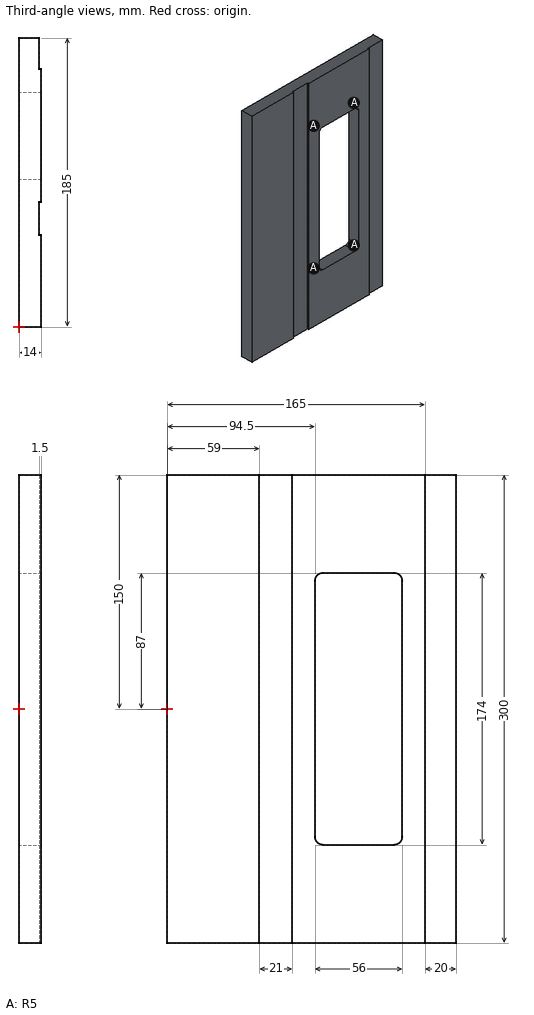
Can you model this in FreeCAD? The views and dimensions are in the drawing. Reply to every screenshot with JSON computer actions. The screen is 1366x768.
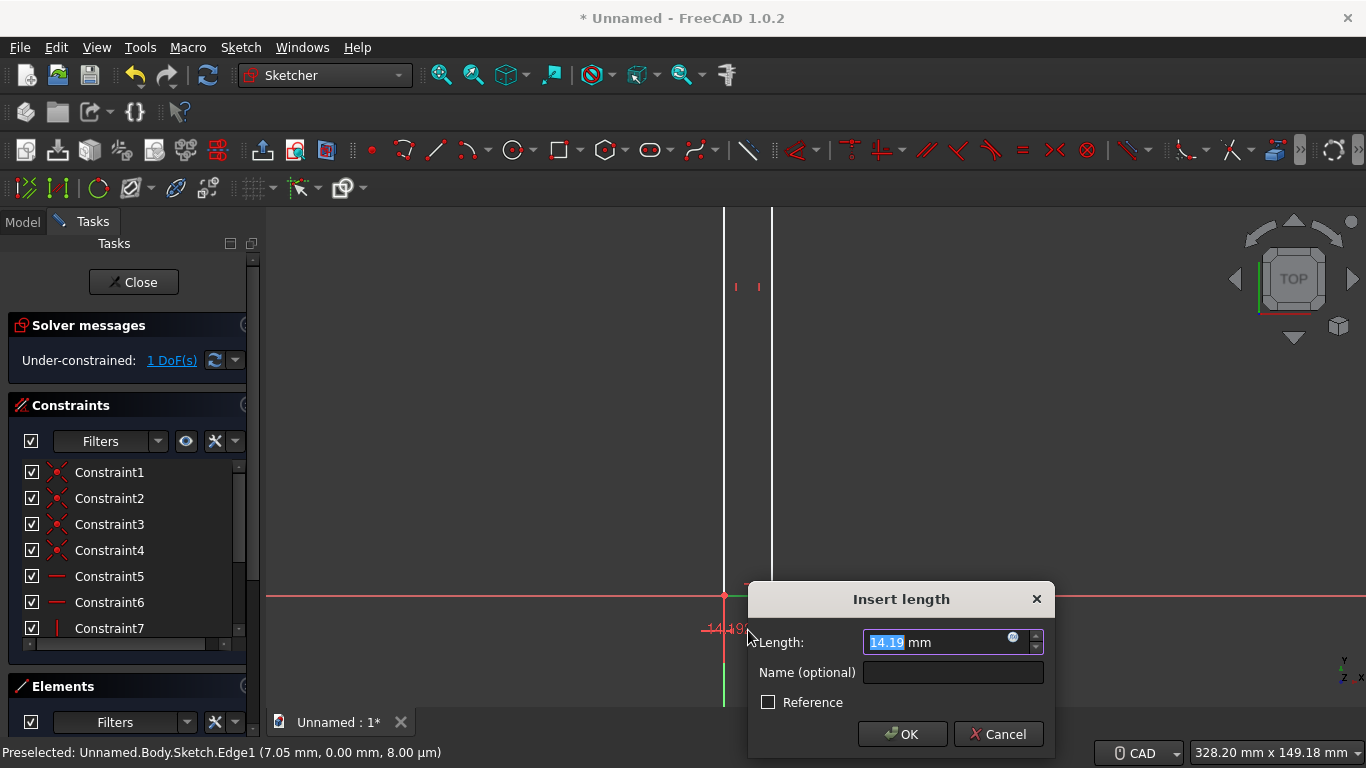
{"action": "type", "text": "14"}
{"action": "key", "text": "Return"}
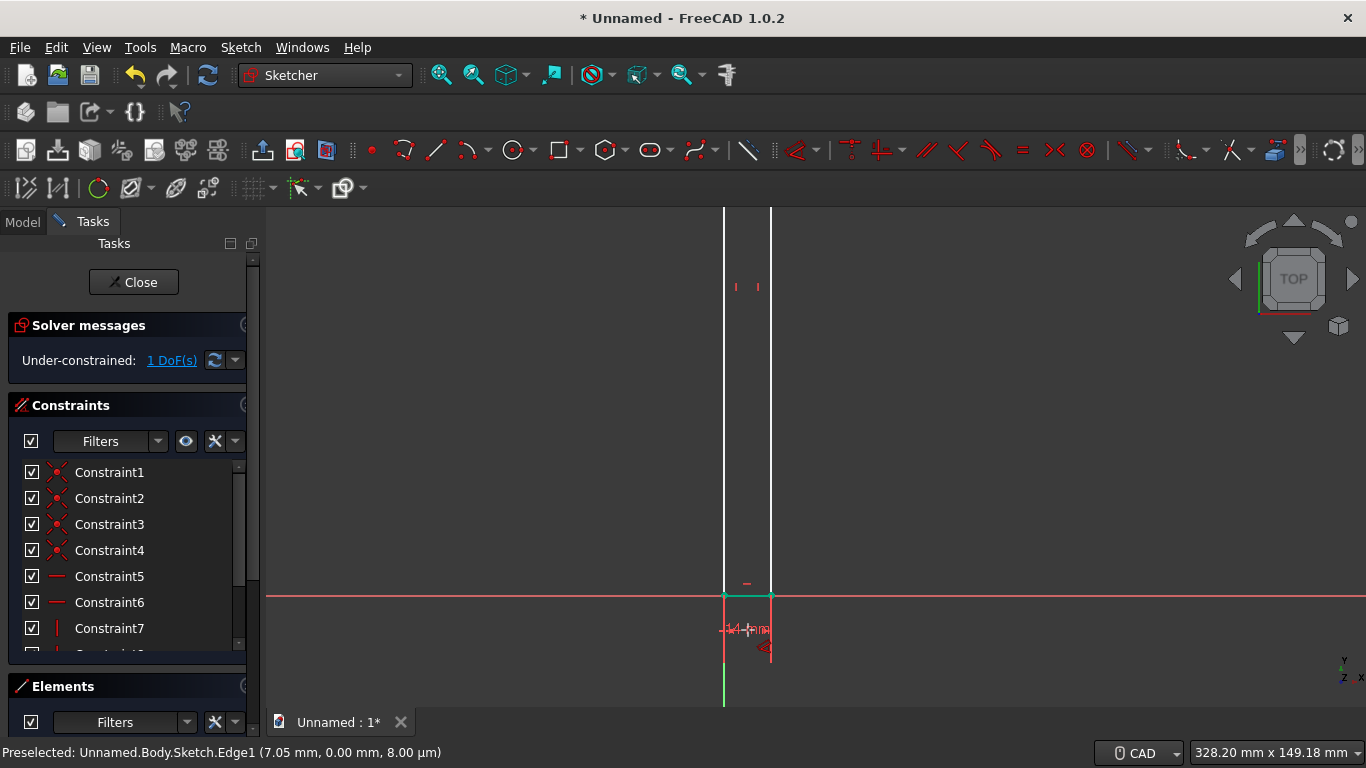
{"action": "left_click", "coordinate": [771, 410]}
{"action": "left_click", "coordinate": [805, 415]}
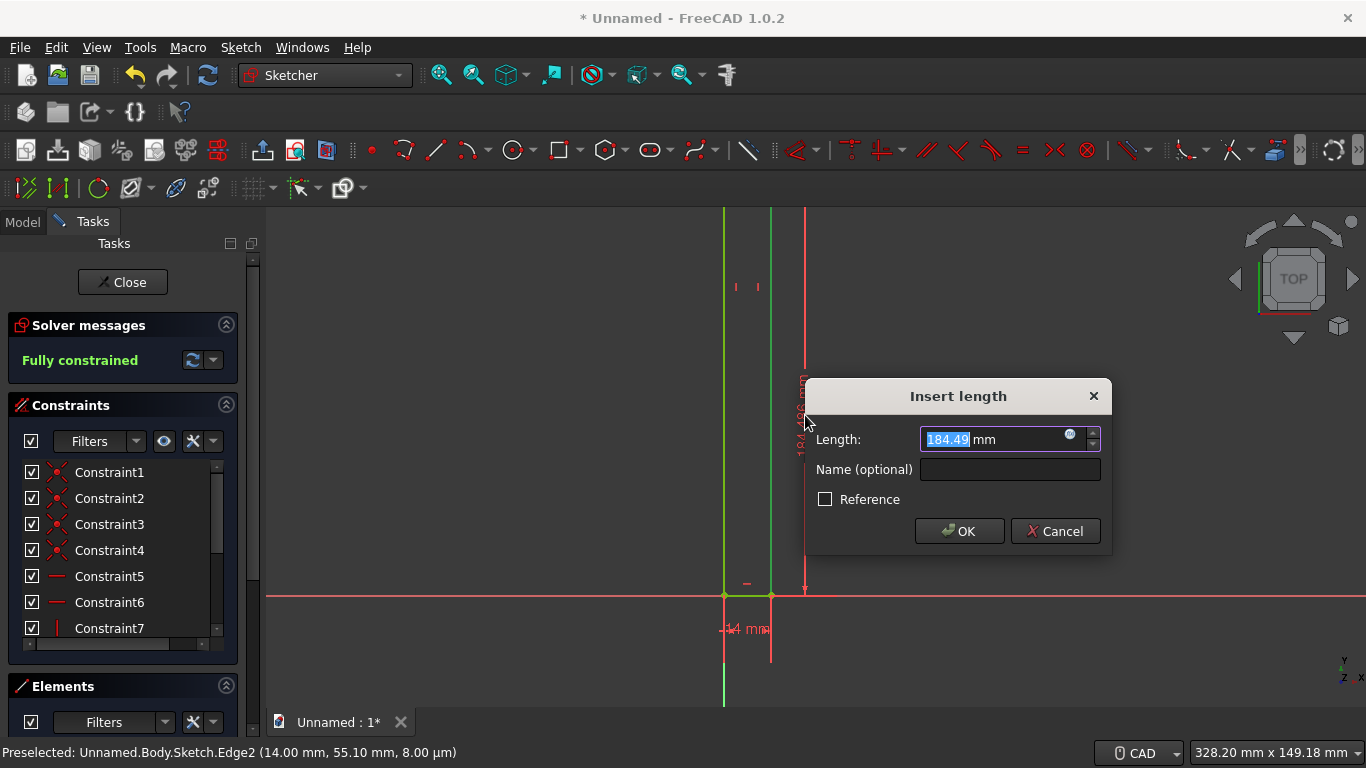
{"action": "type", "text": "185"}
{"action": "key", "text": "Return"}
{"action": "key", "text": "Escape"}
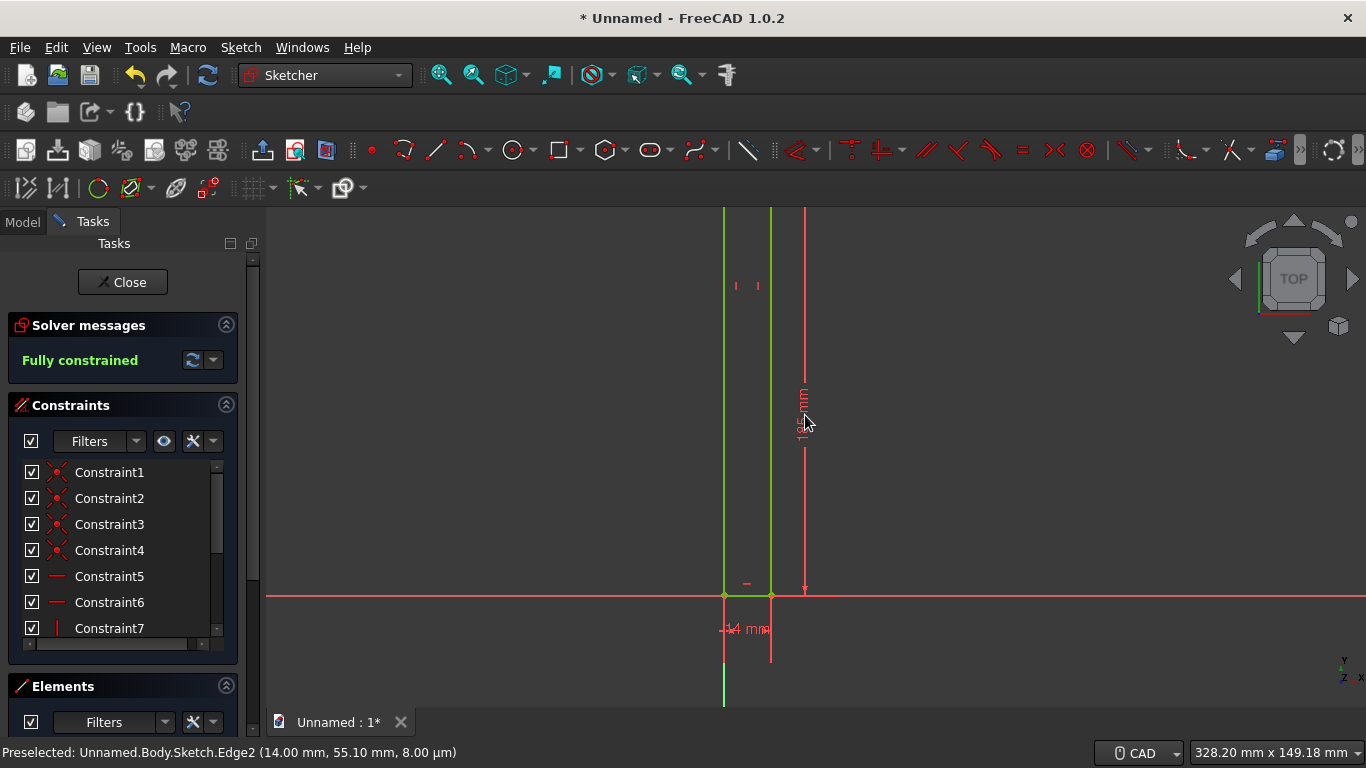
{"action": "left_click", "coordinate": [123, 282]}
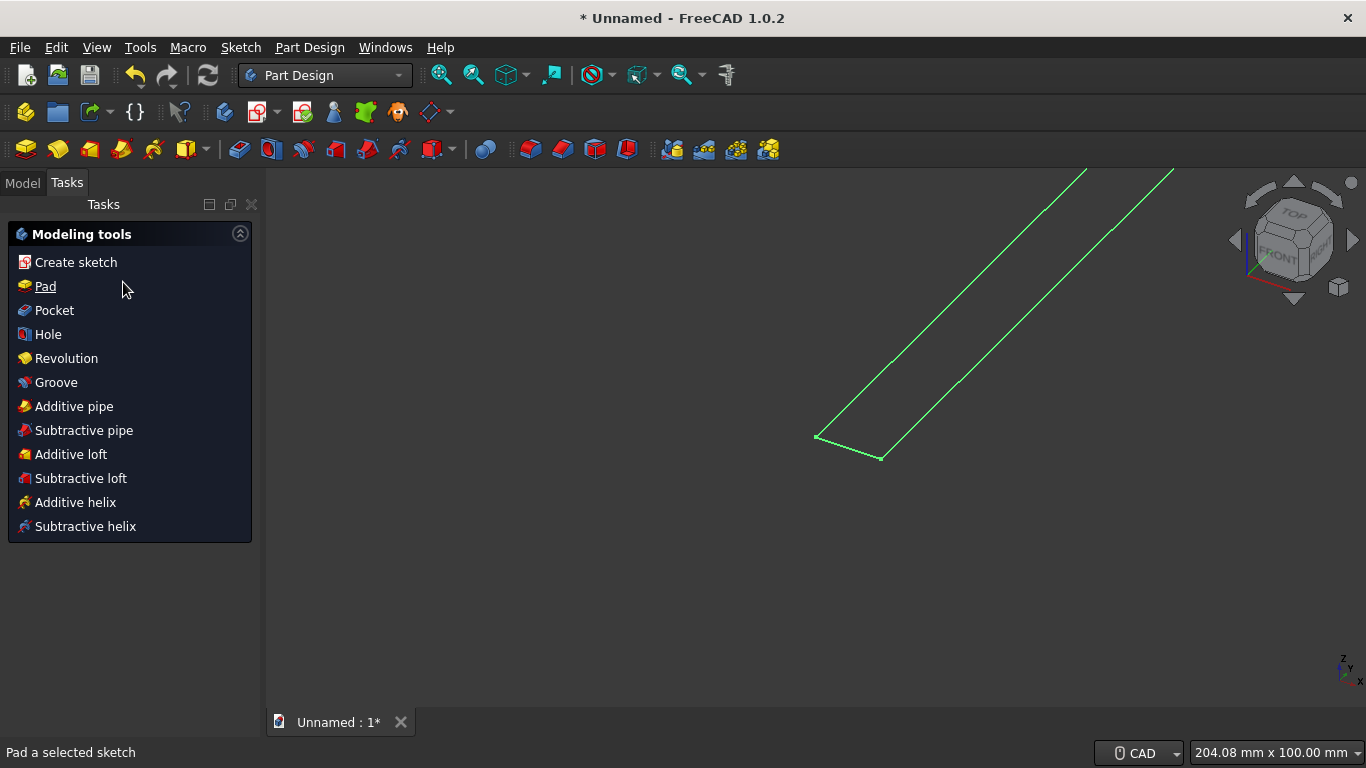
{"action": "left_click", "coordinate": [26, 150]}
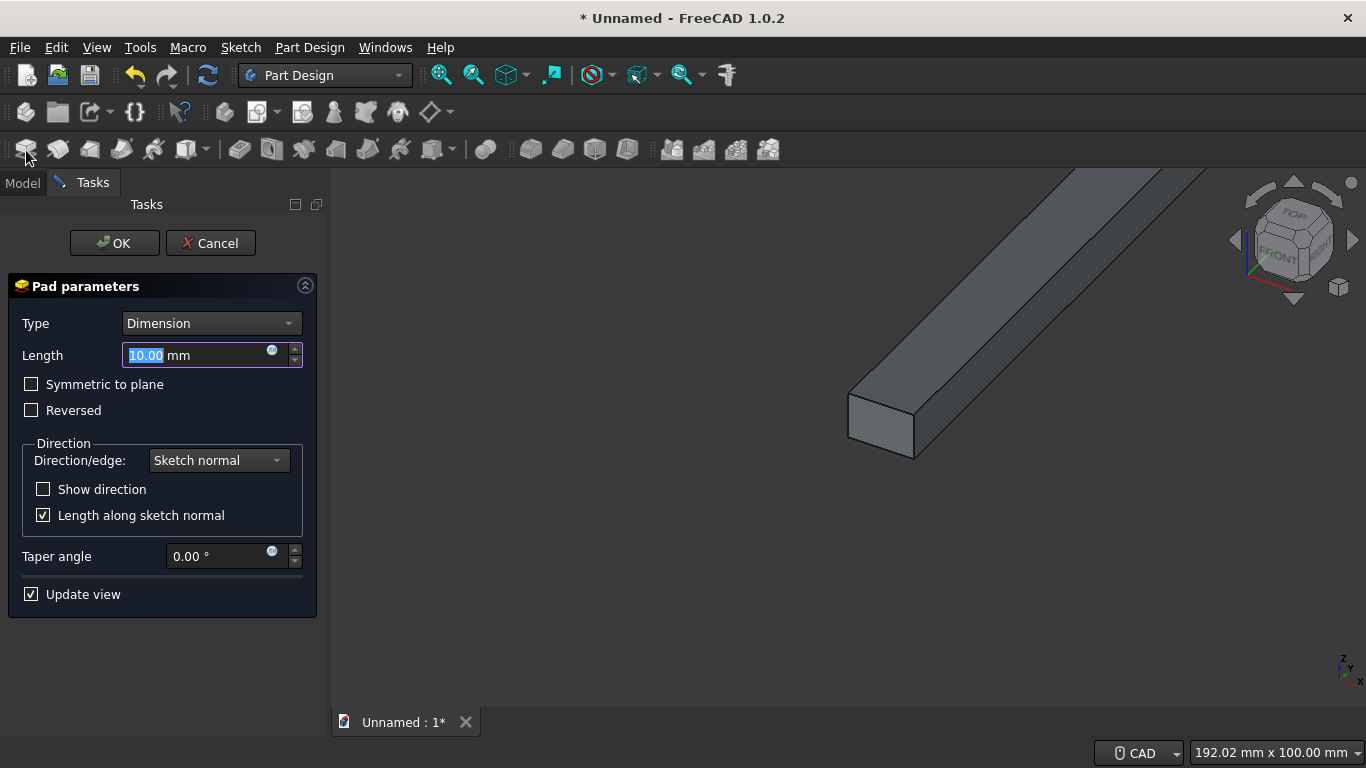
{"action": "type", "text": "300"}
{"action": "key", "text": "Tab"}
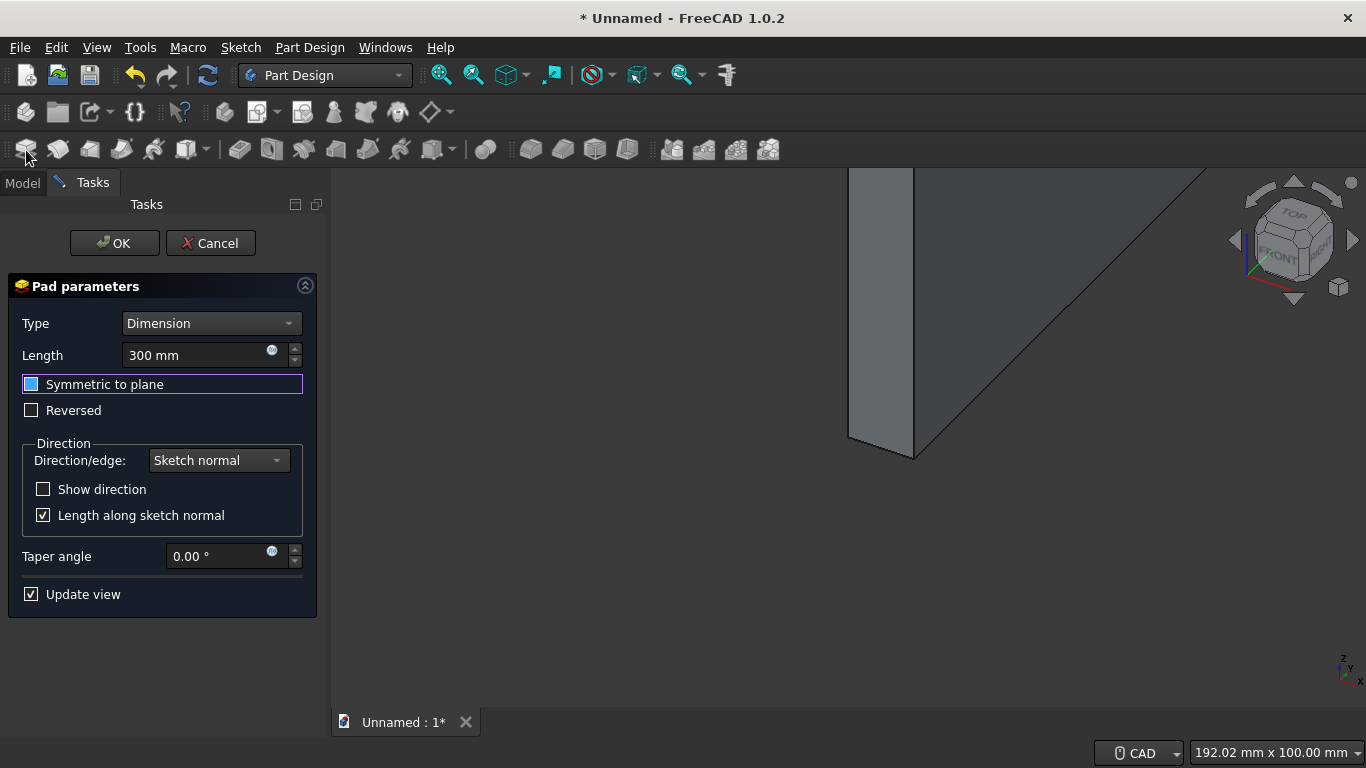
{"action": "left_click", "coordinate": [30, 384]}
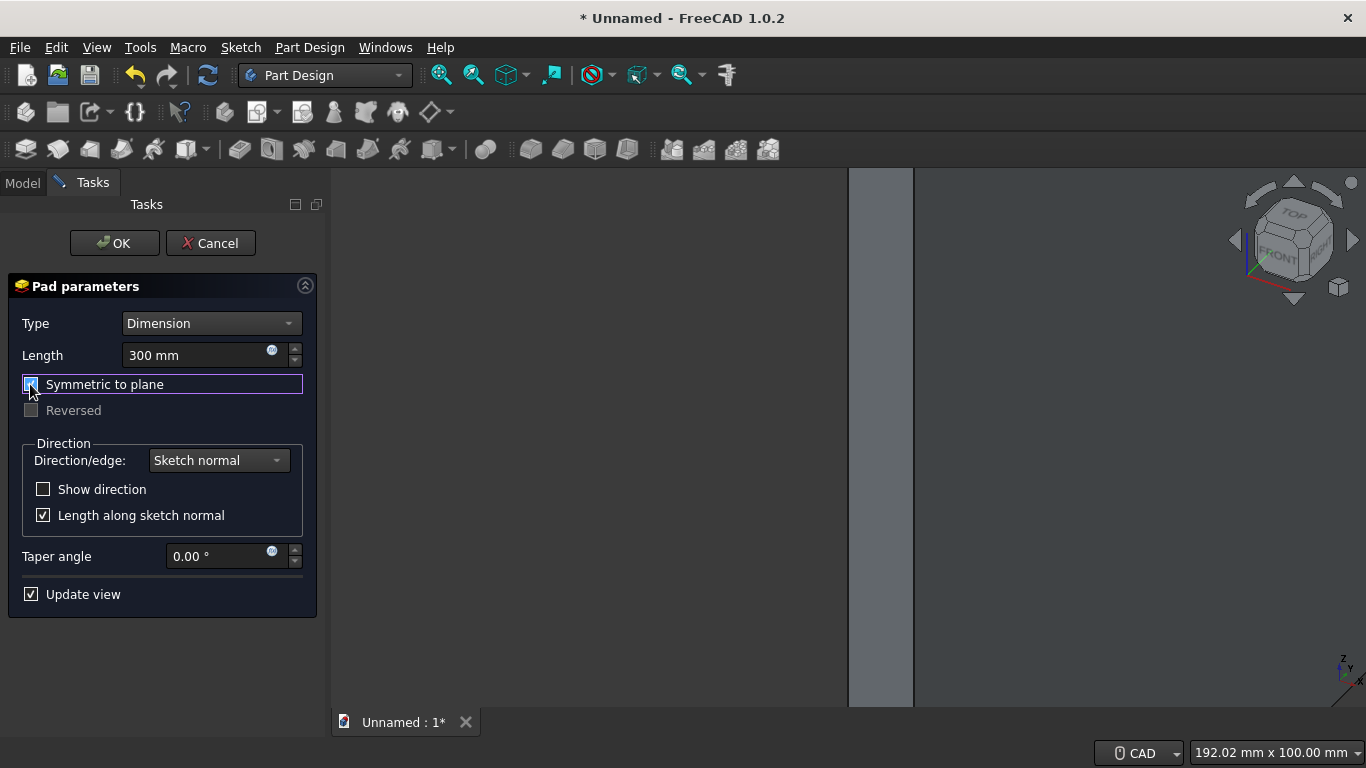
{"action": "left_click", "coordinate": [115, 243]}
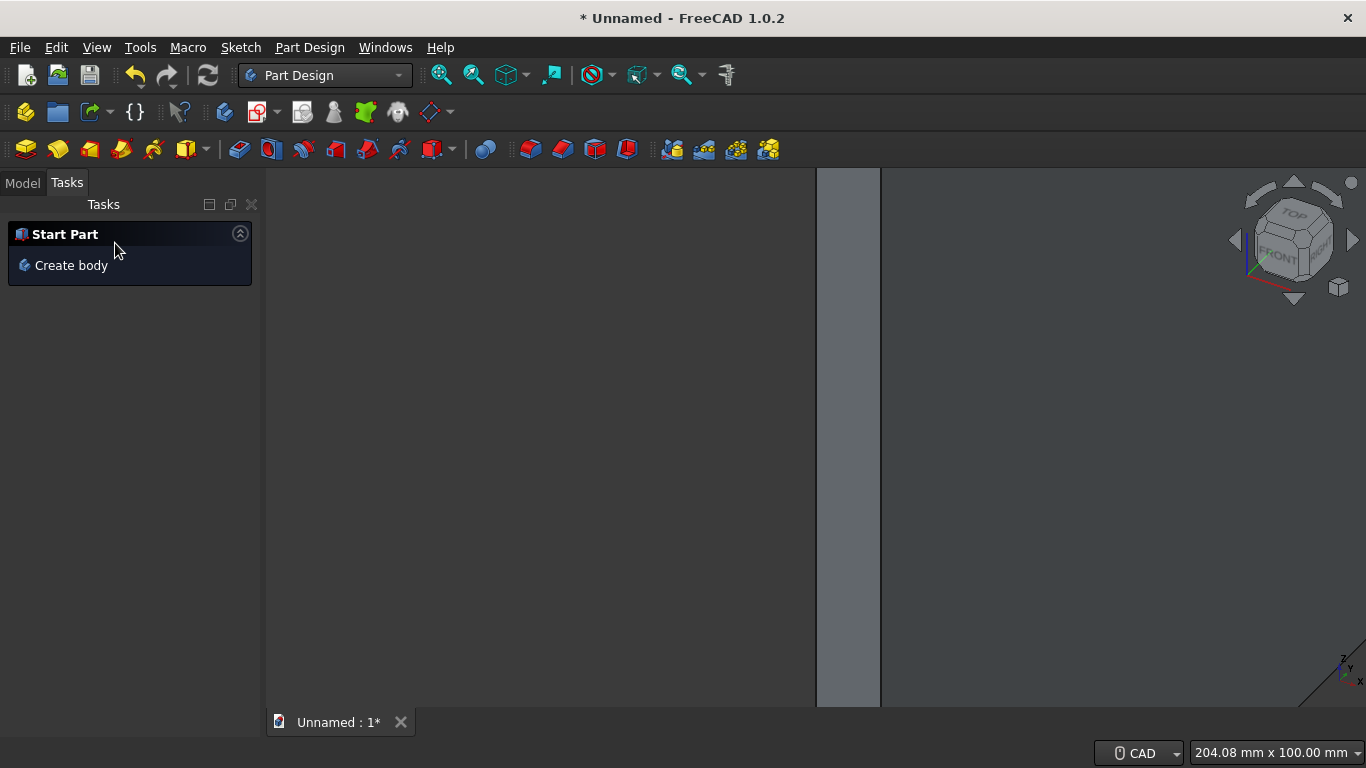
{"action": "key", "text": "v f"}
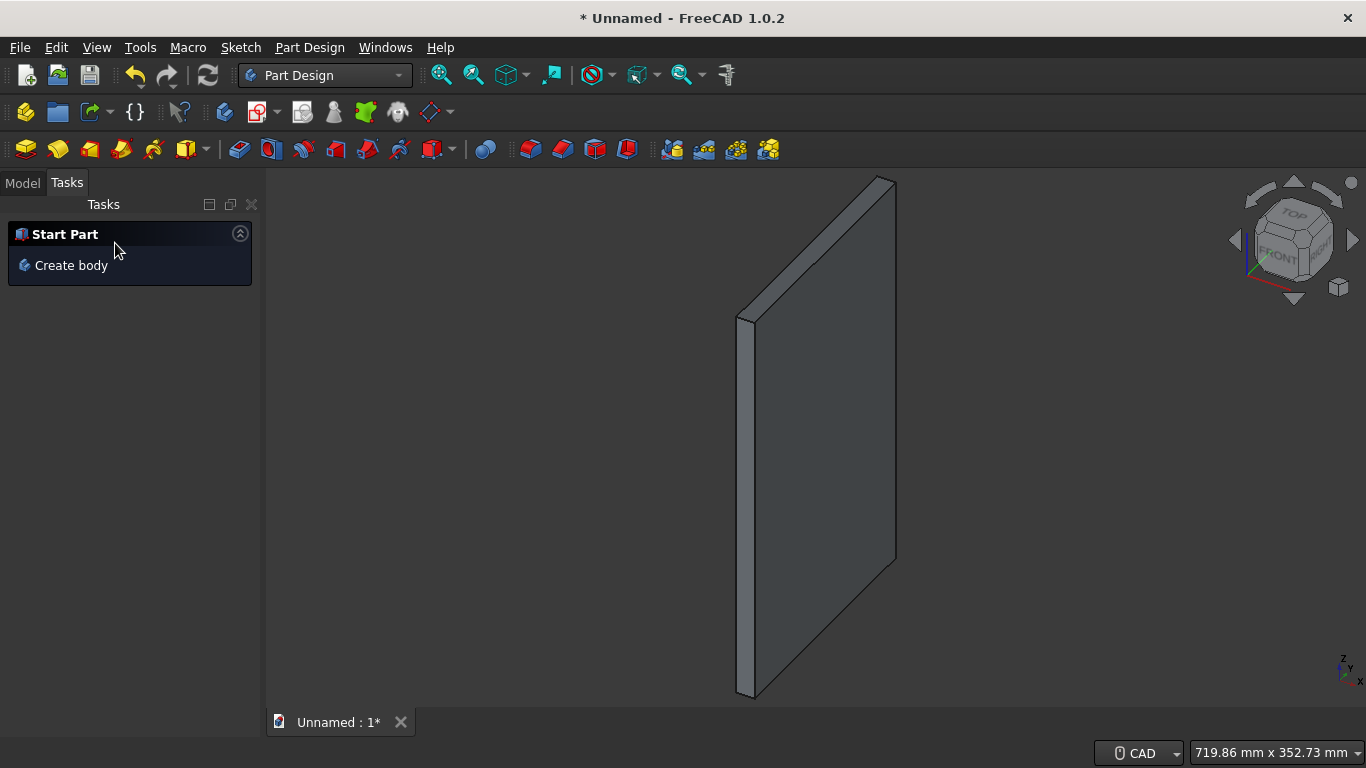
{"action": "left_click", "coordinate": [825, 386]}